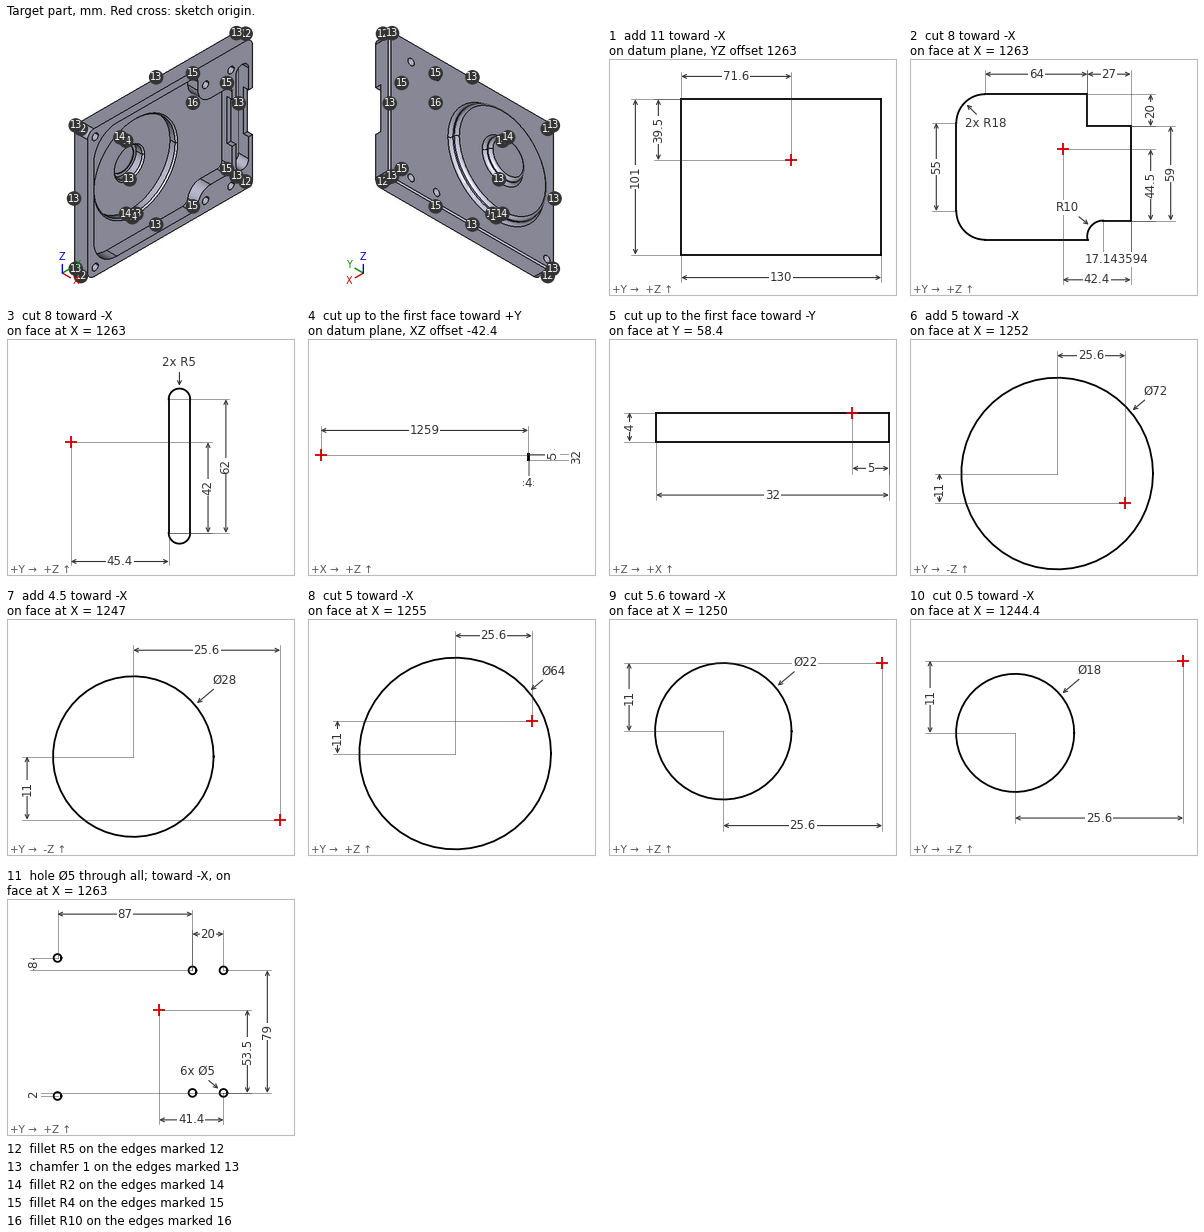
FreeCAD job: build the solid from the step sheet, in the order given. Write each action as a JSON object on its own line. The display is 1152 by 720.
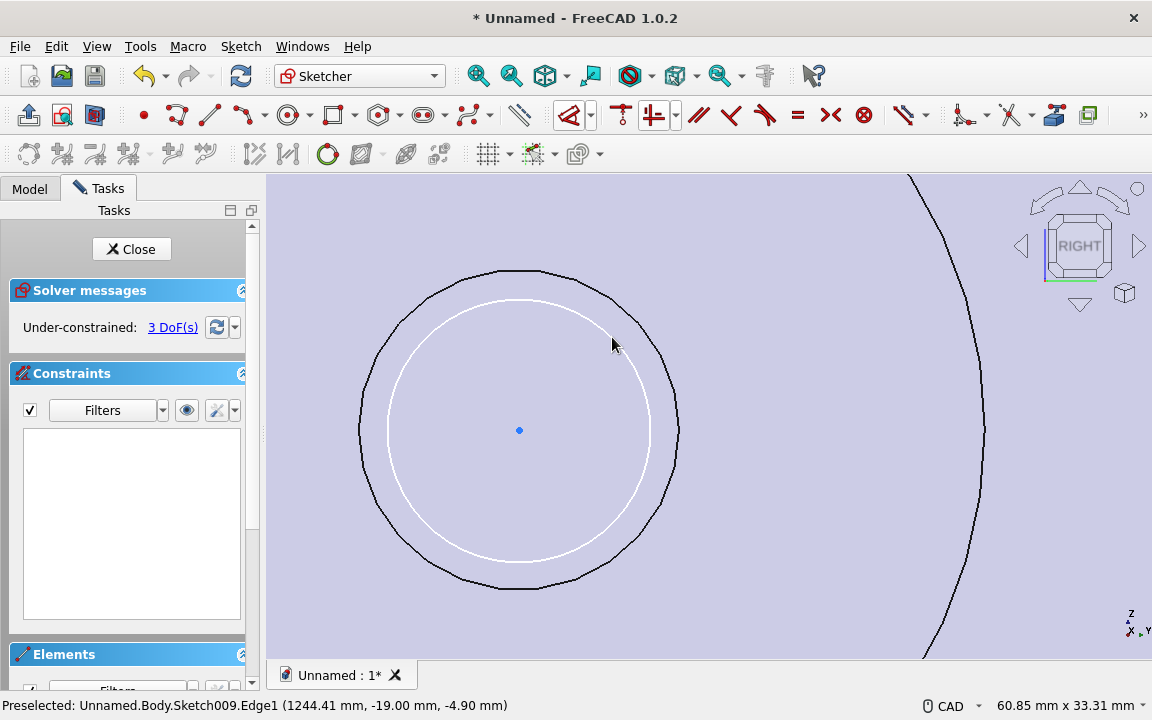
{"action": "left_click", "coordinate": [612, 338]}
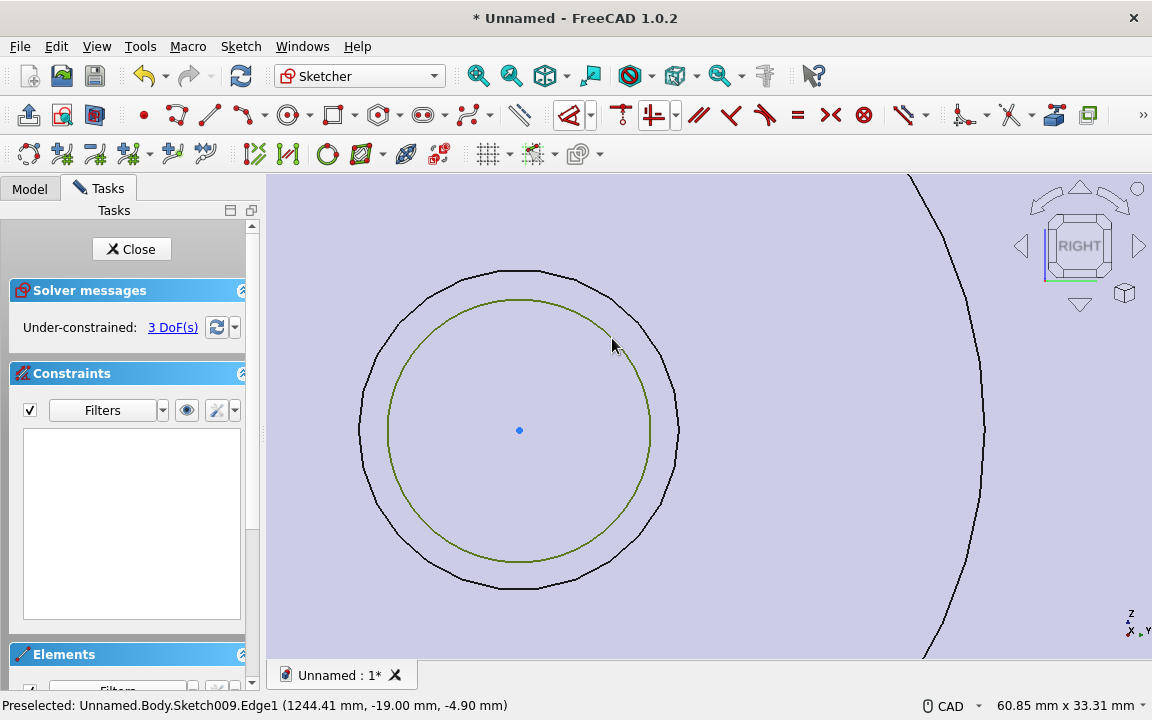
{"action": "left_click", "coordinate": [590, 116]}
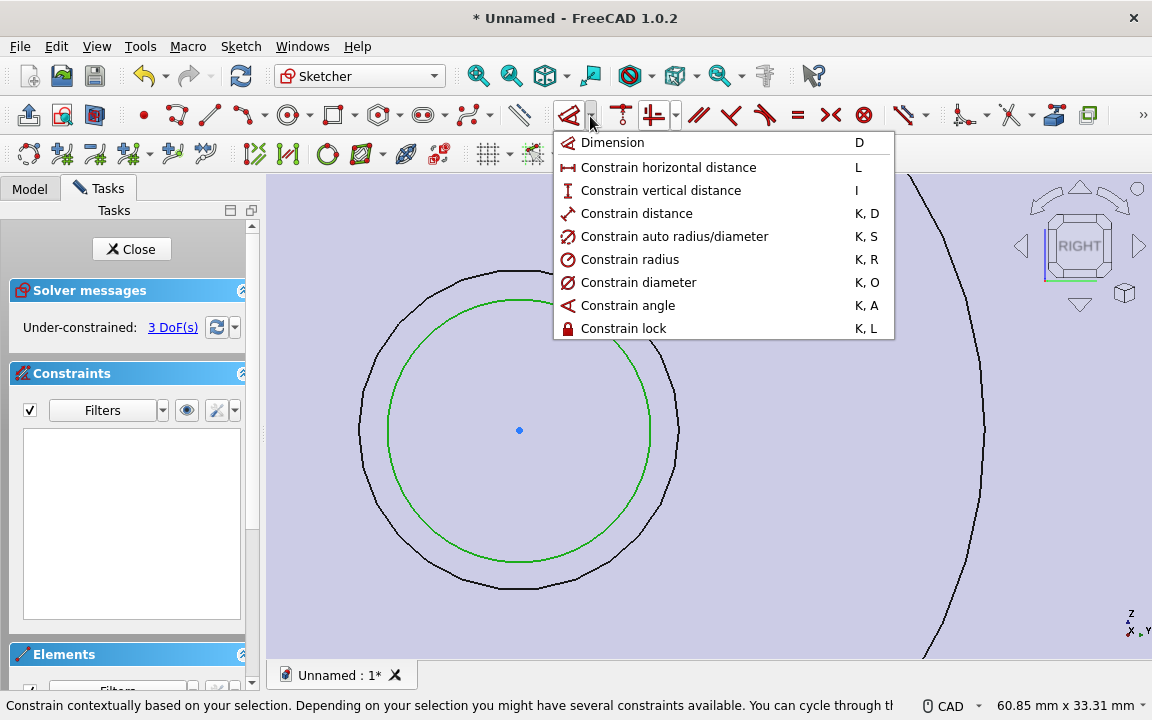
{"action": "left_click", "coordinate": [724, 282]}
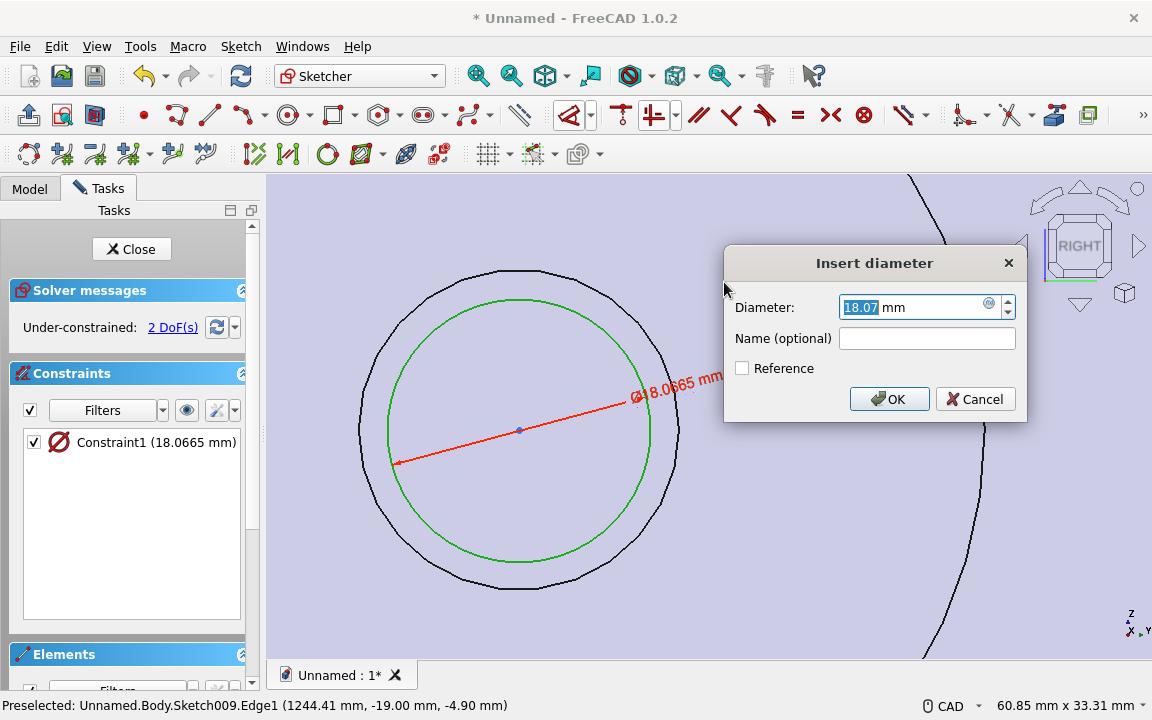
{"action": "type", "text": "18"}
{"action": "key", "text": "Return"}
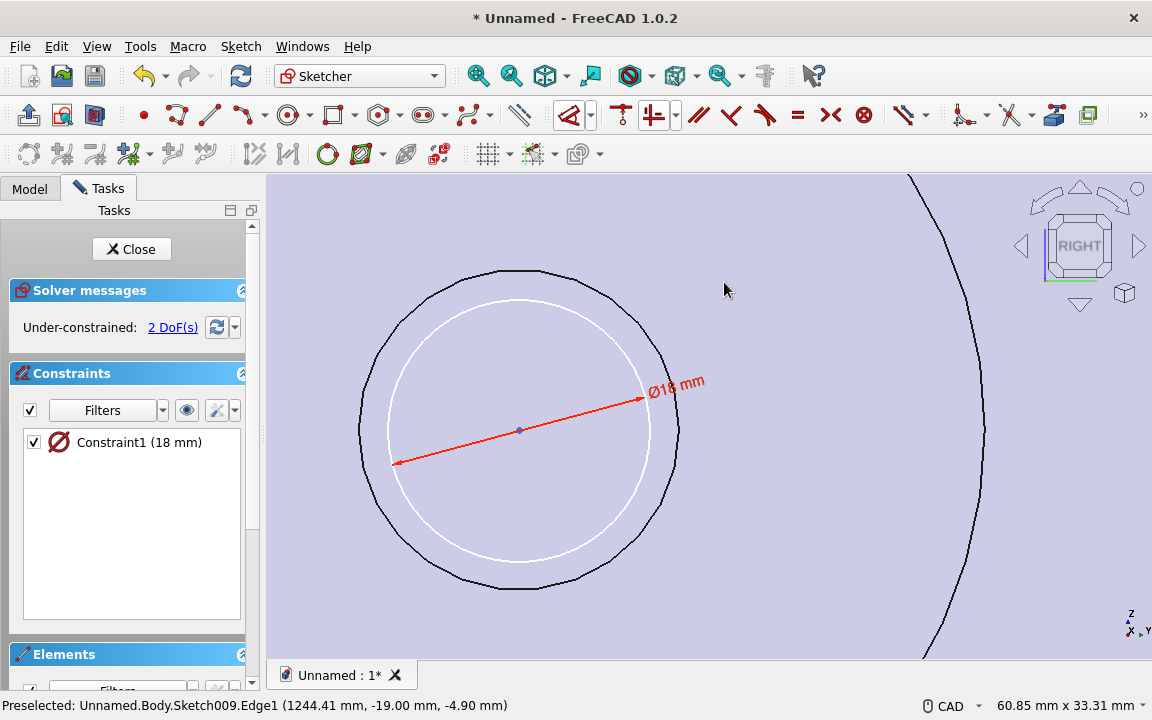
{"action": "left_click", "coordinate": [519, 431]}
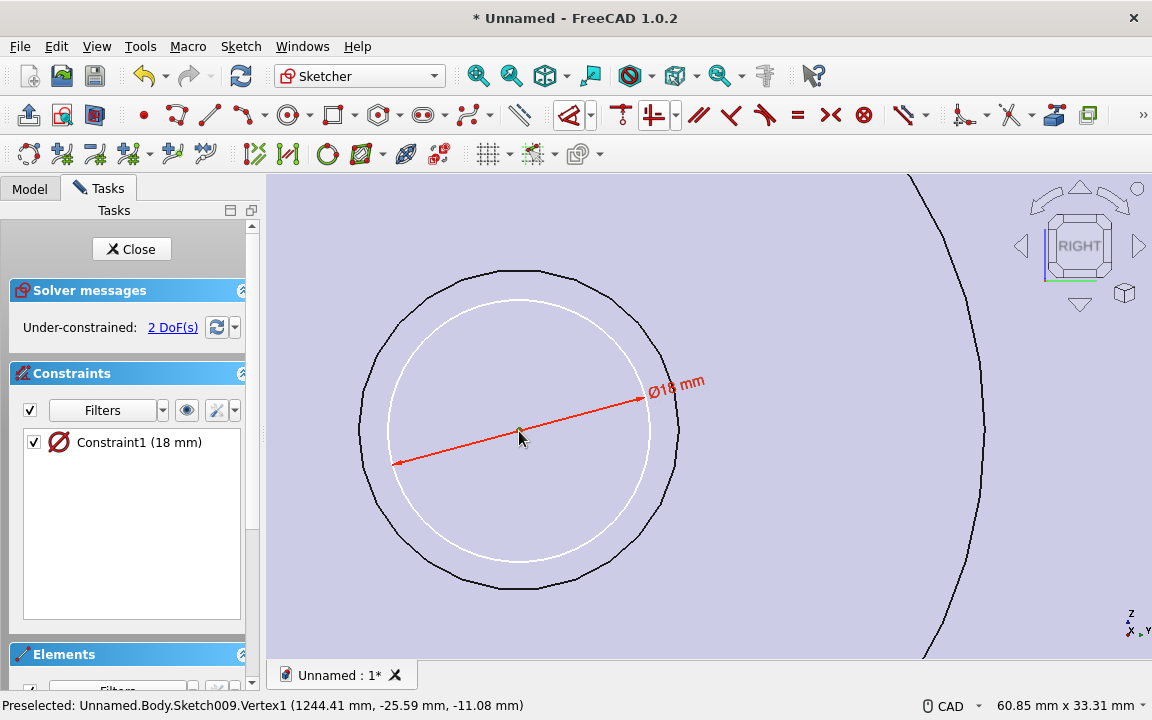
{"action": "left_click", "coordinate": [590, 116]}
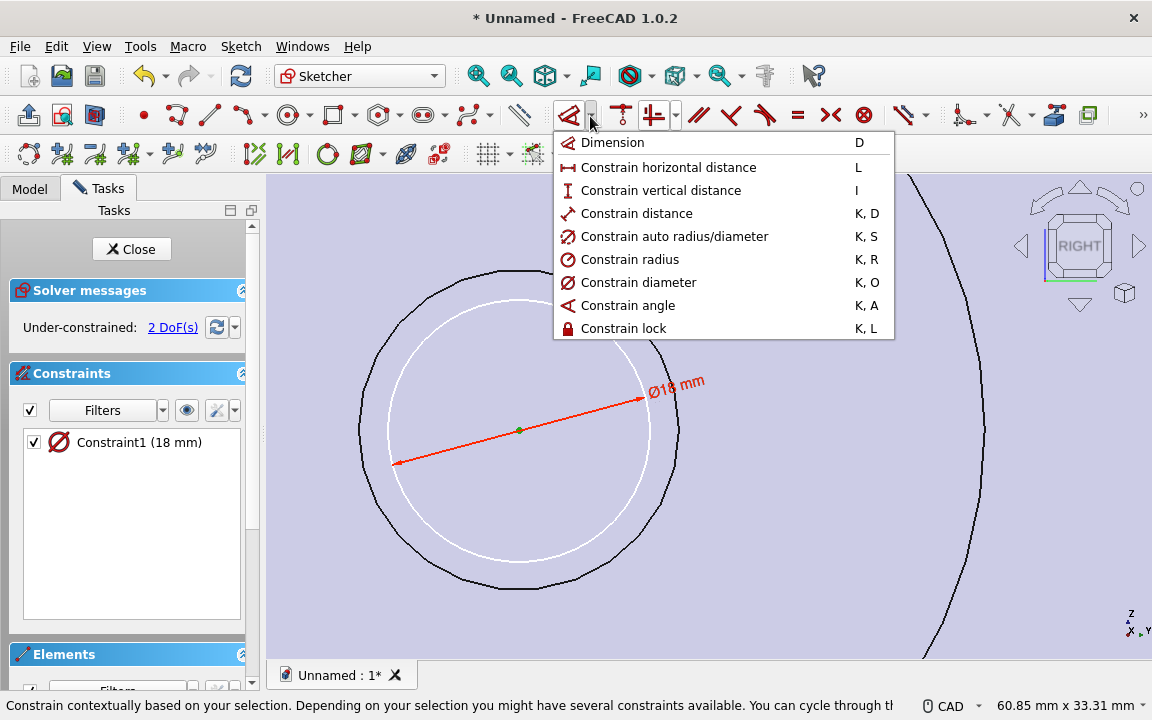
{"action": "left_click", "coordinate": [724, 190]}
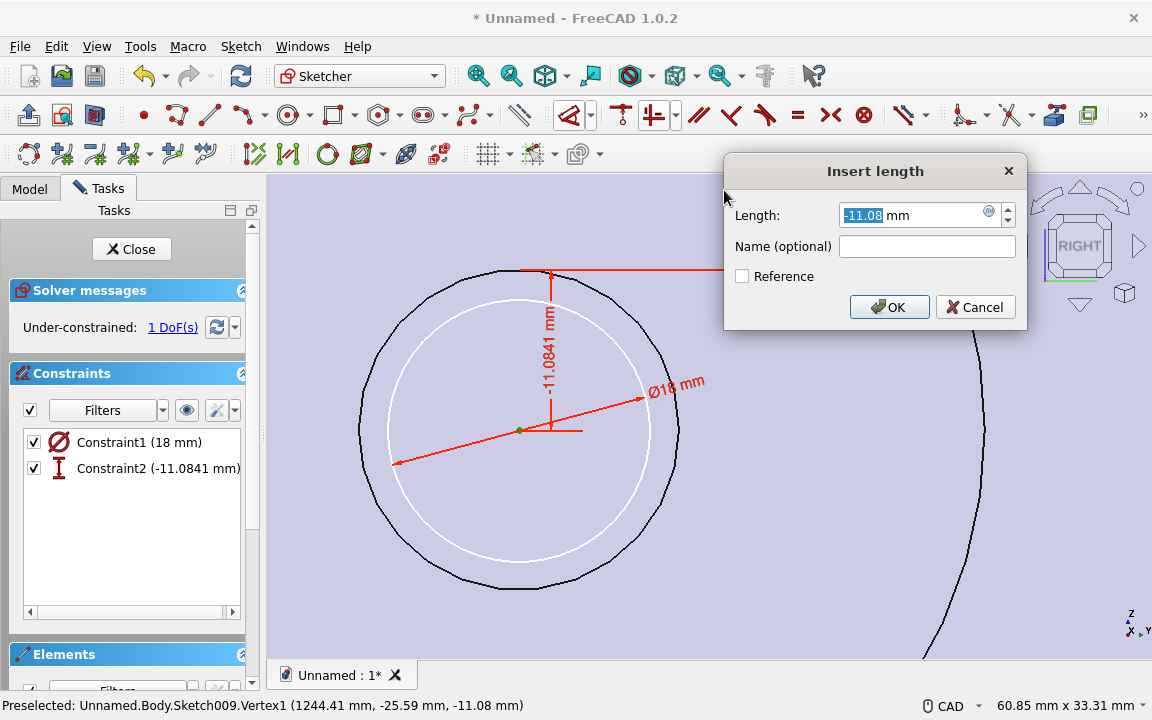
{"action": "type", "text": "-11"}
{"action": "key", "text": "Return"}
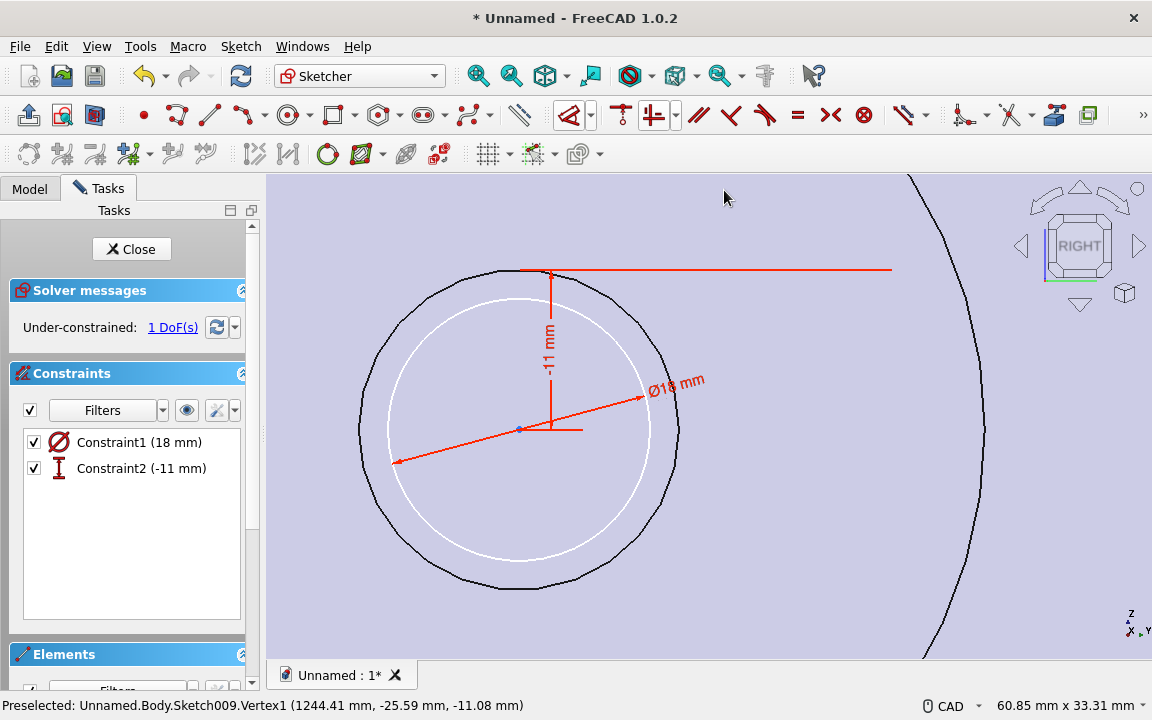
{"action": "left_click", "coordinate": [519, 430]}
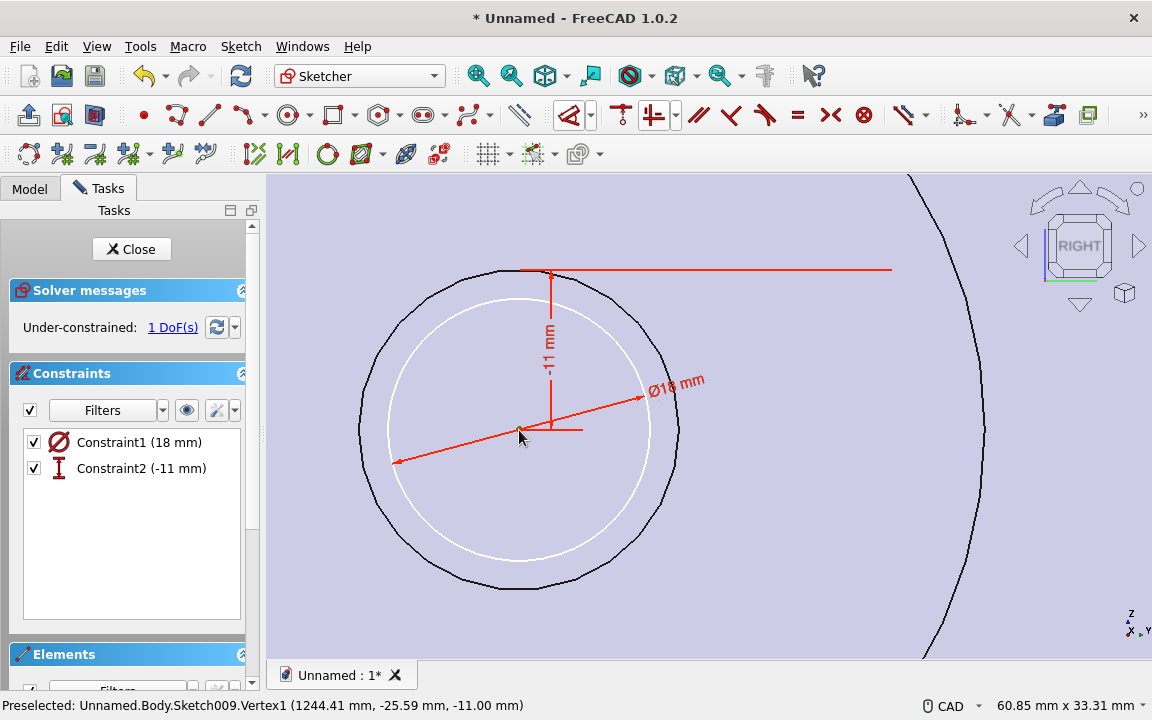
{"action": "key", "text": "l"}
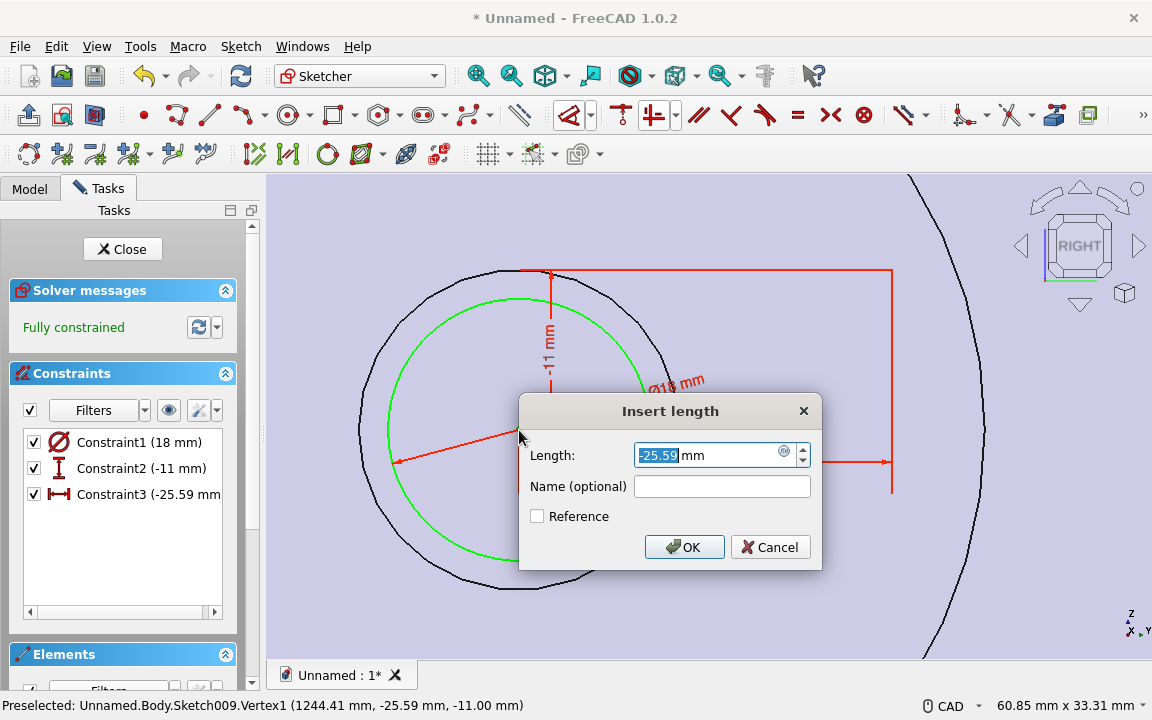
{"action": "type", "text": "-25.6"}
{"action": "key", "text": "Return"}